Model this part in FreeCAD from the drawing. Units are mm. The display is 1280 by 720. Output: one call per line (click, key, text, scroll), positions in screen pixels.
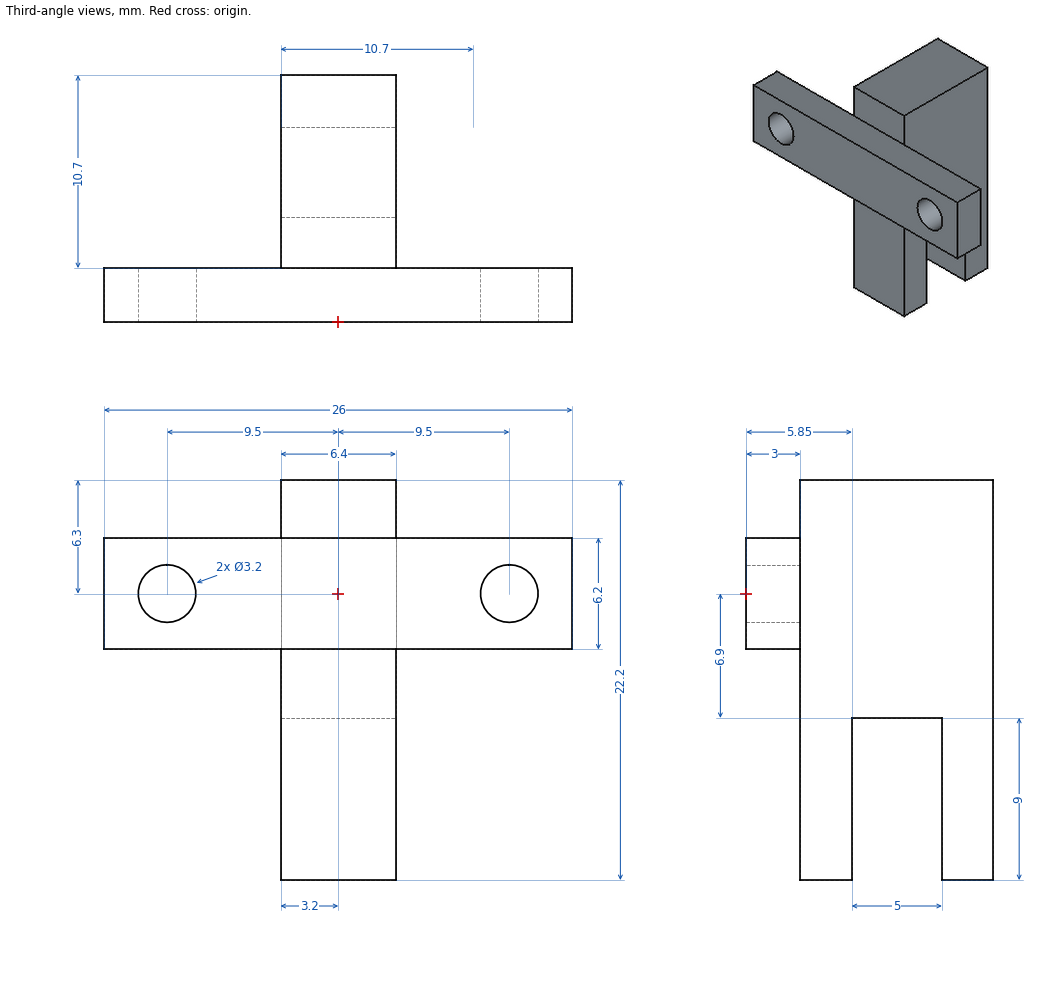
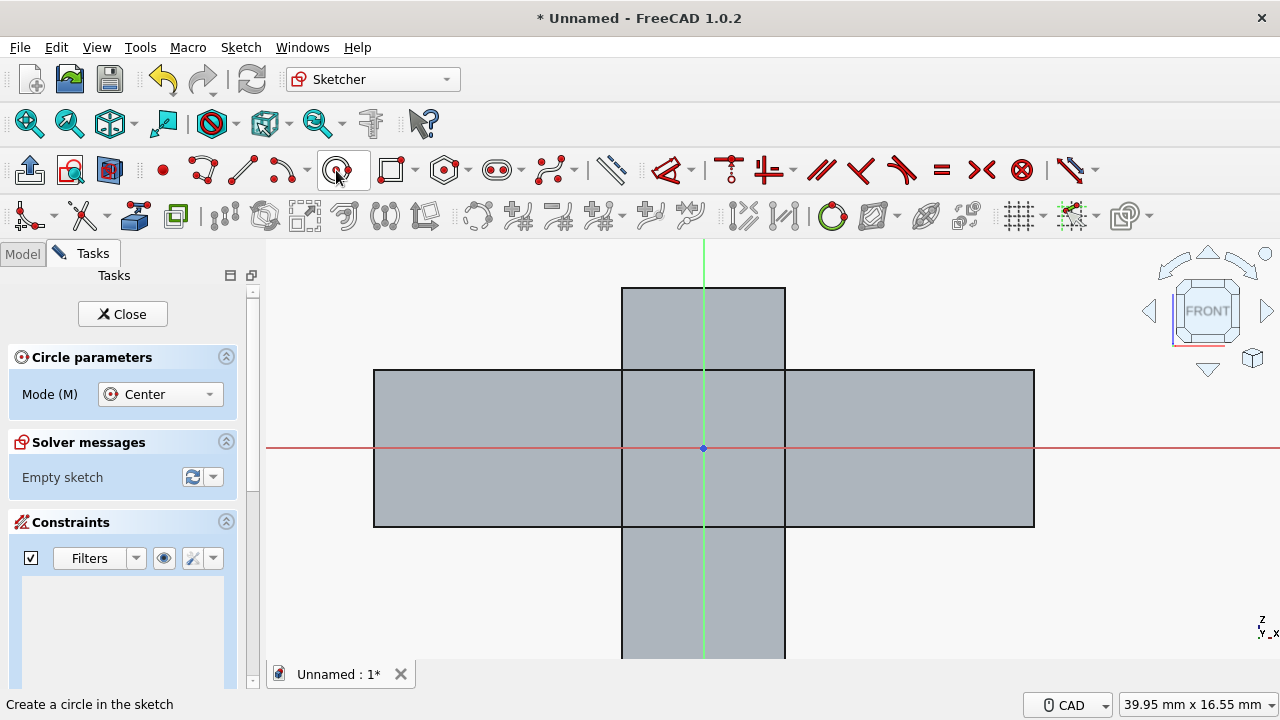
click(463, 448)
move(491, 419)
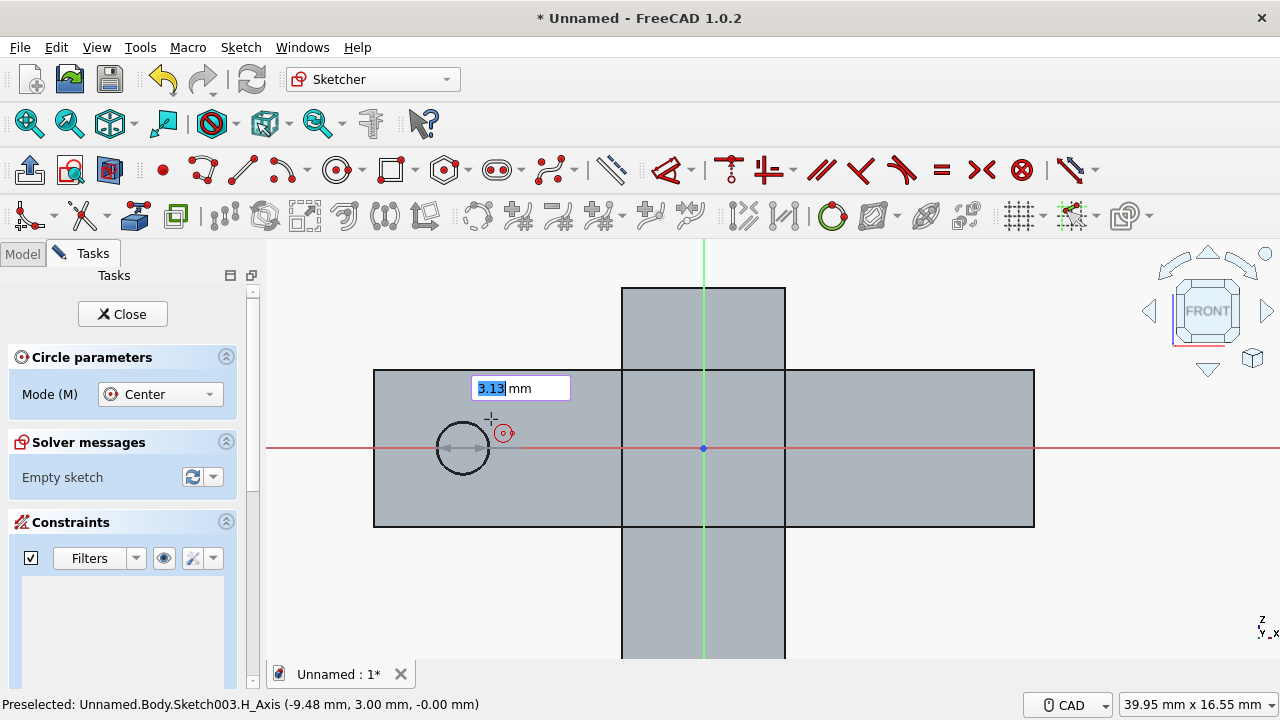
text(3.2)
key(Return)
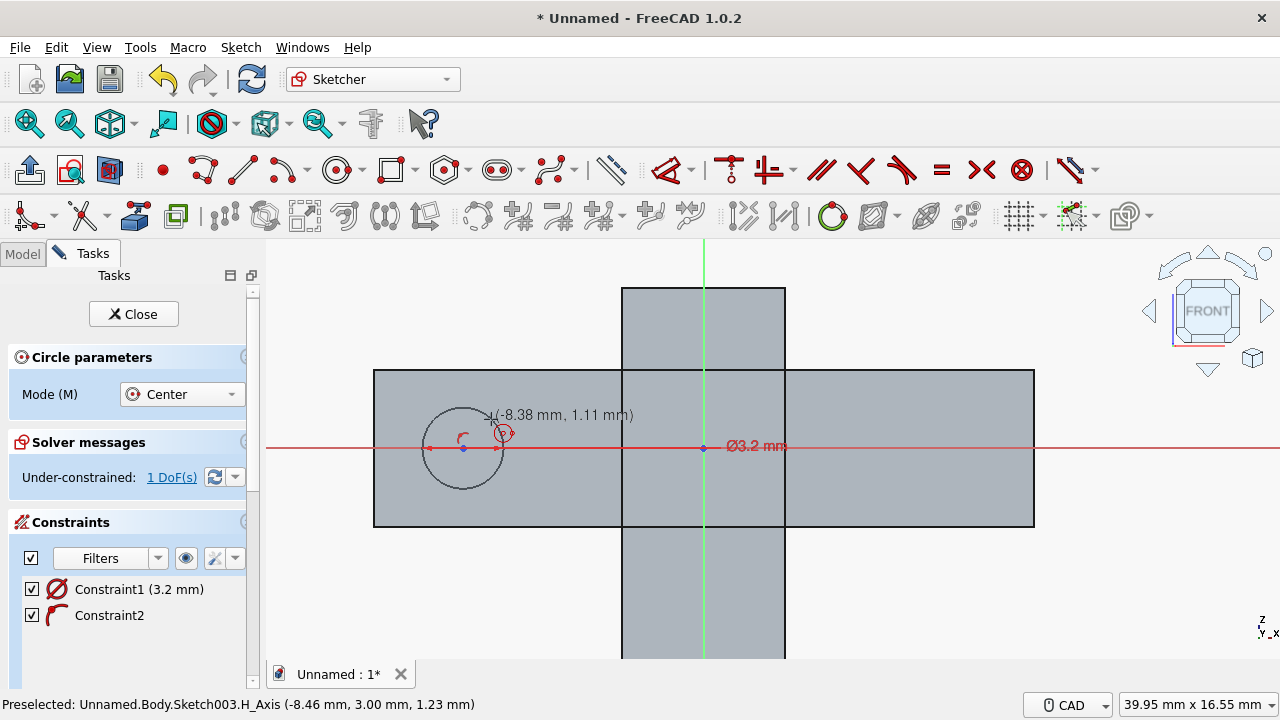
click(945, 448)
move(973, 419)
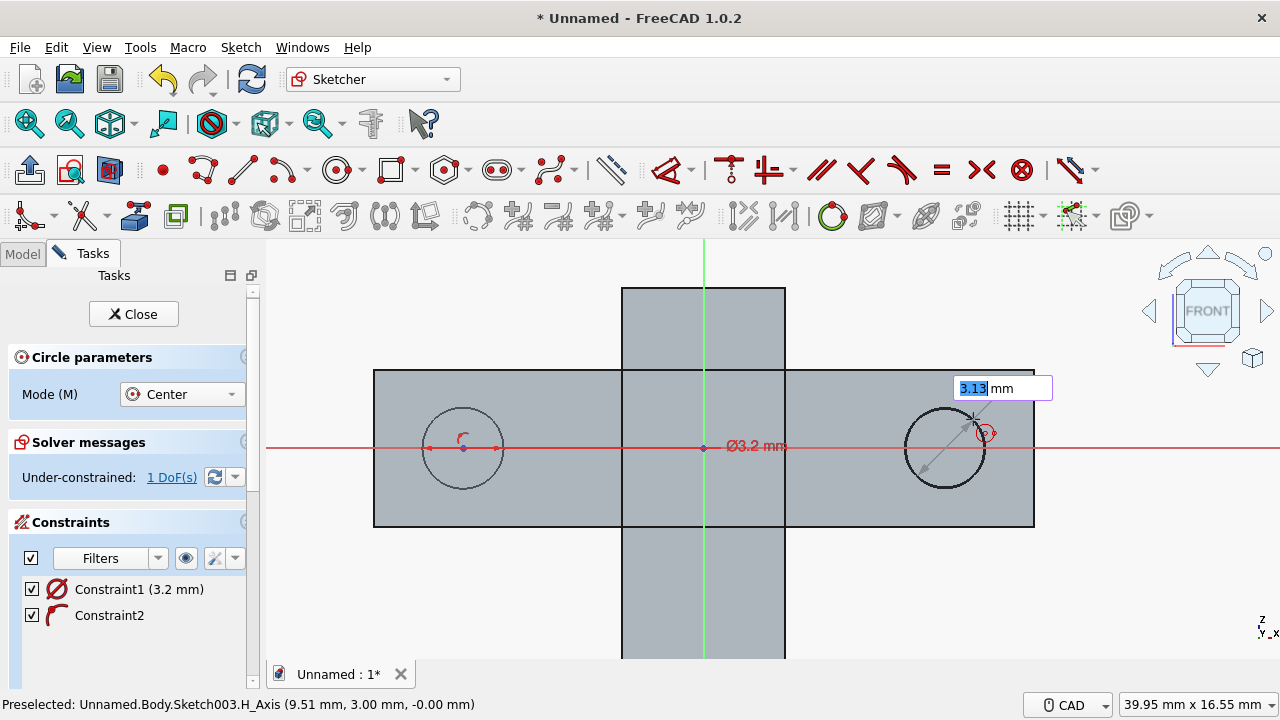
text(3.2)
key(Return)
key(Escape)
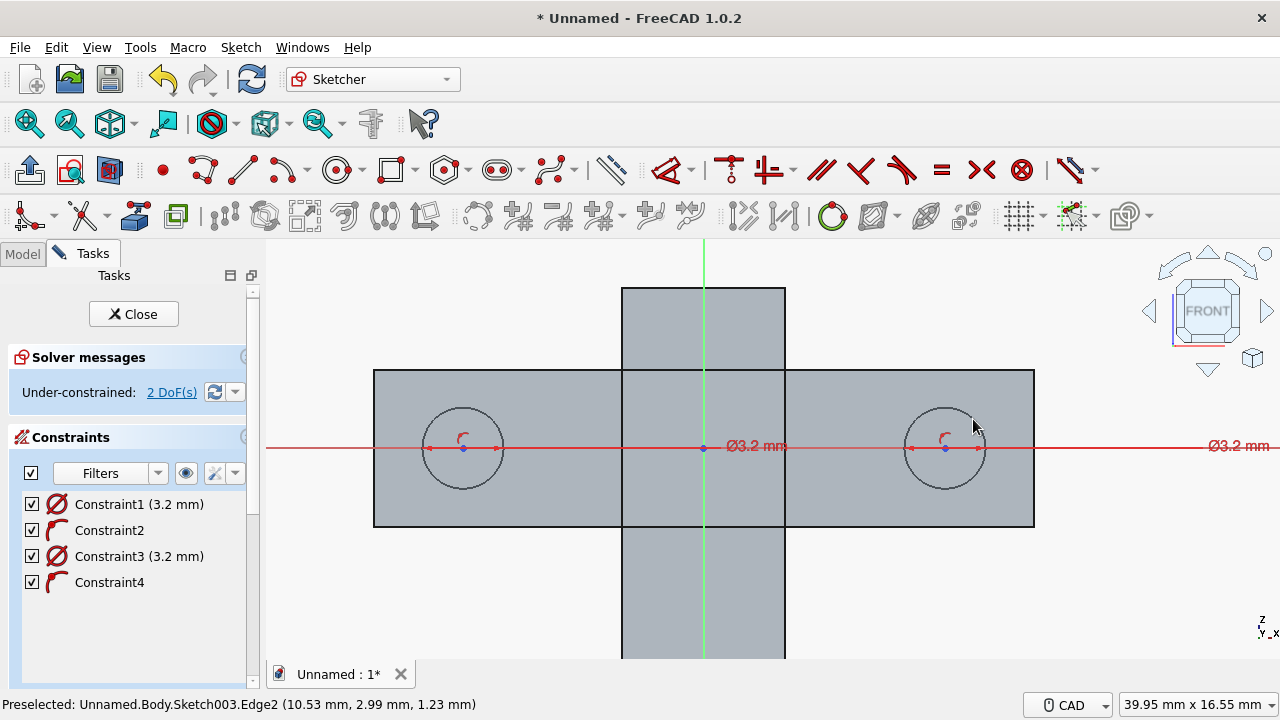
key(d)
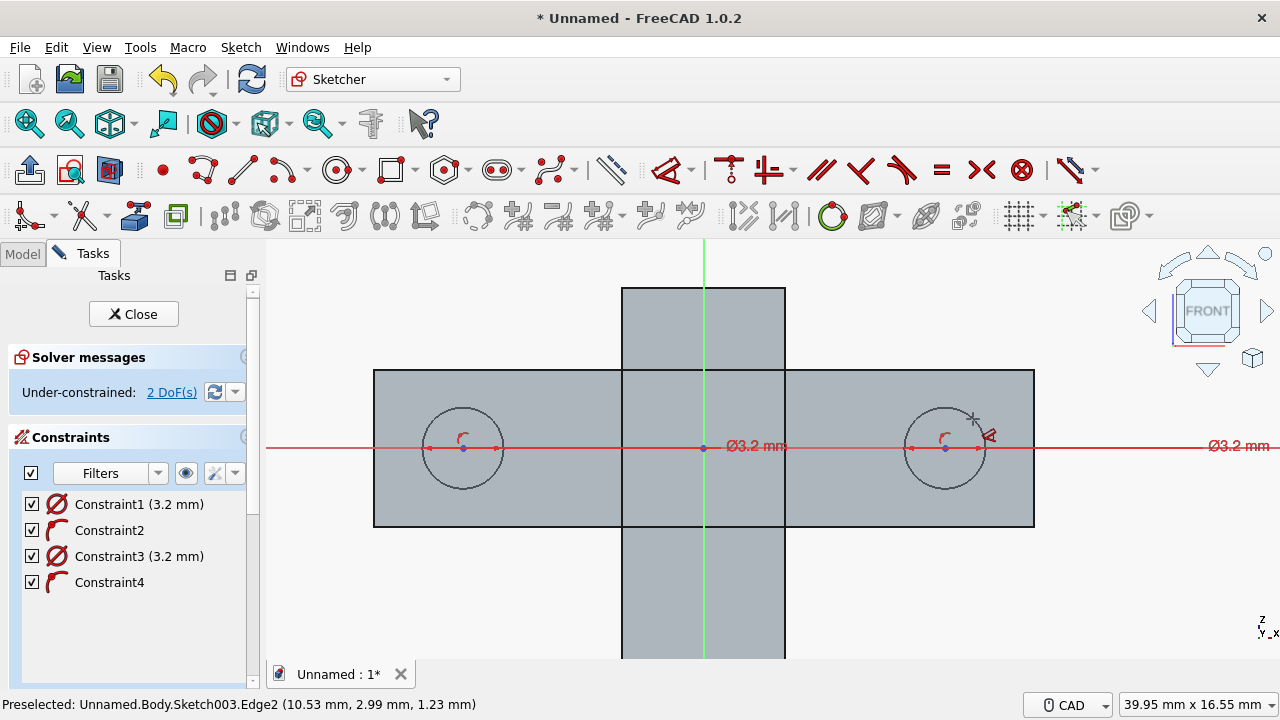
click(463, 448)
click(583, 482)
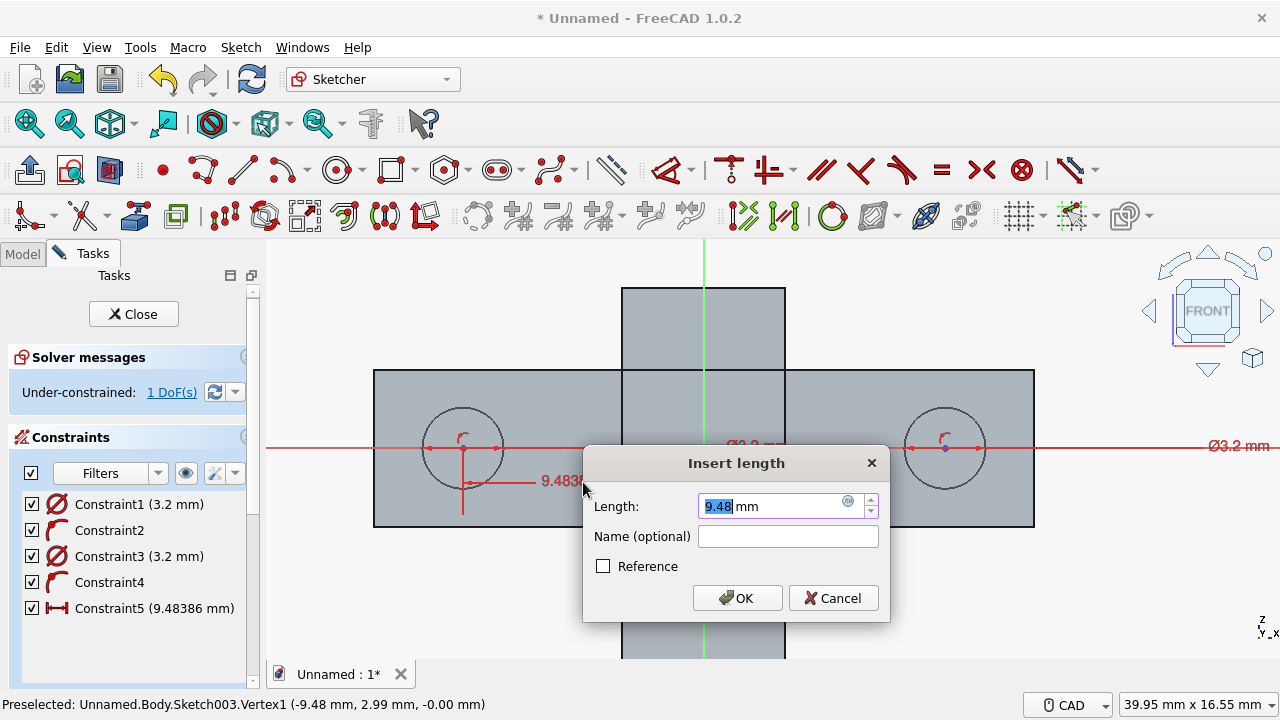
text(9.5)
key(Return)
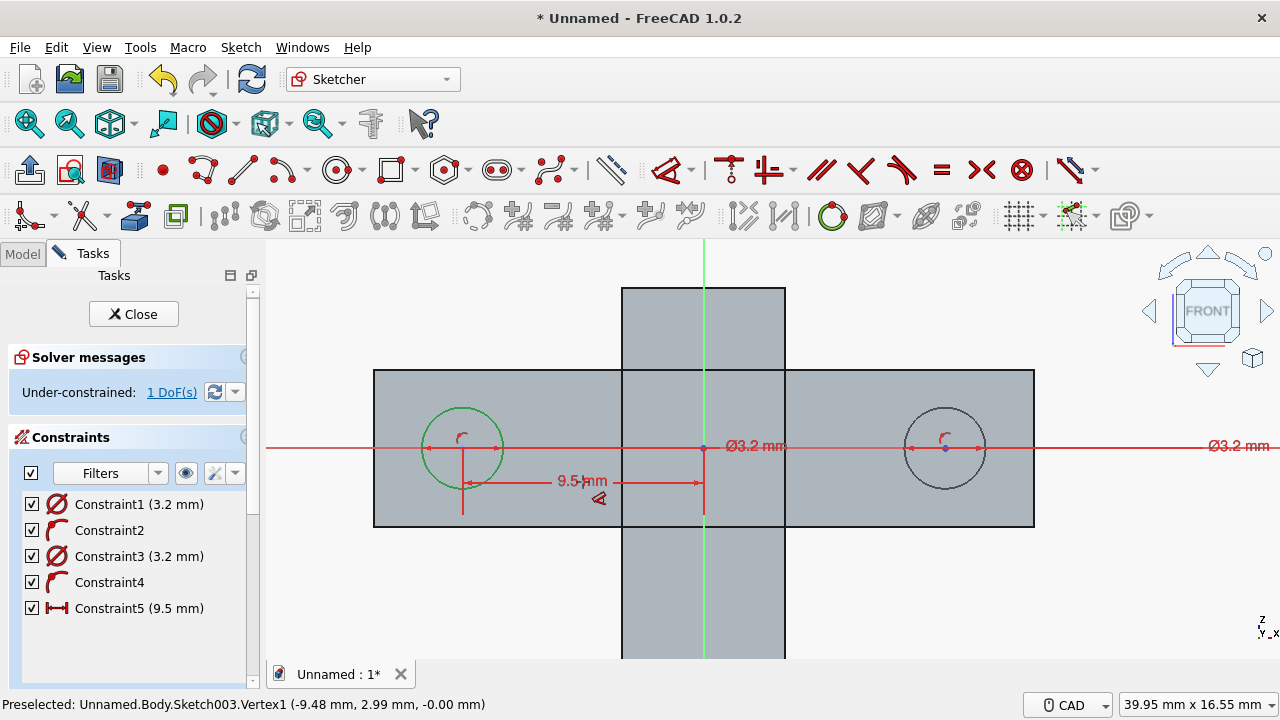
click(945, 448)
click(824, 482)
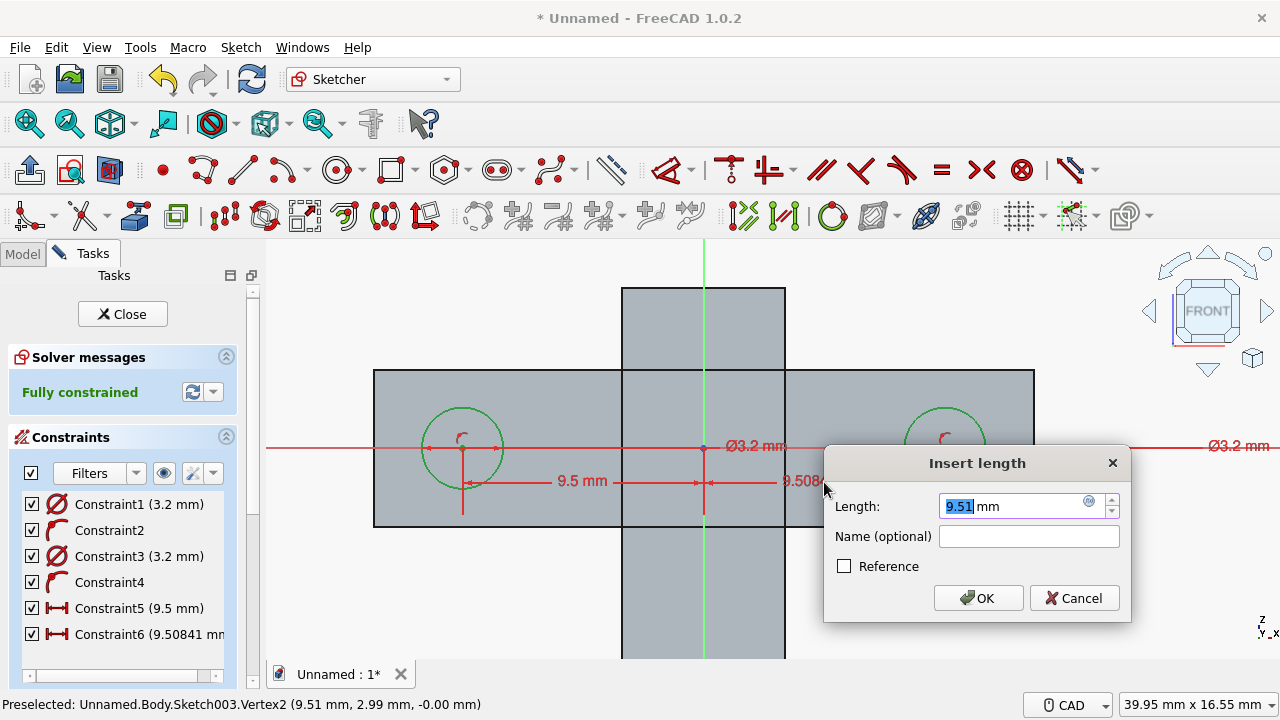
text(9.5)
key(Return)
key(Escape)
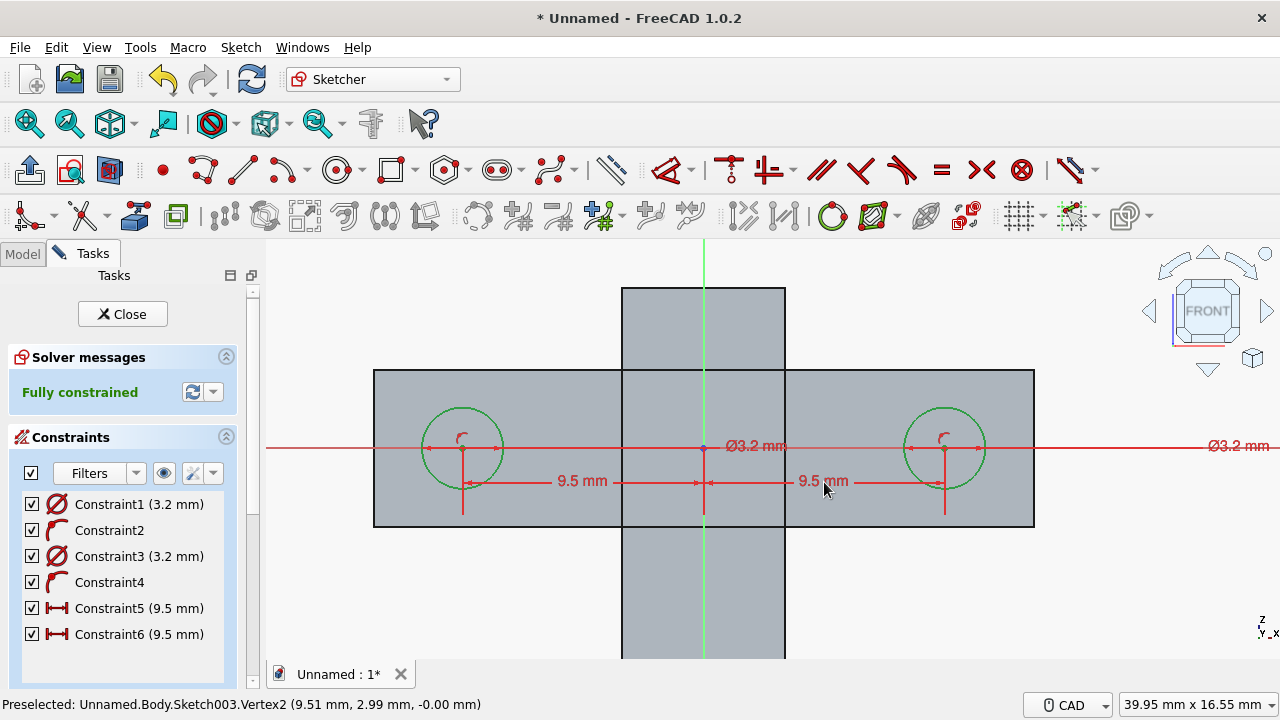
click(123, 314)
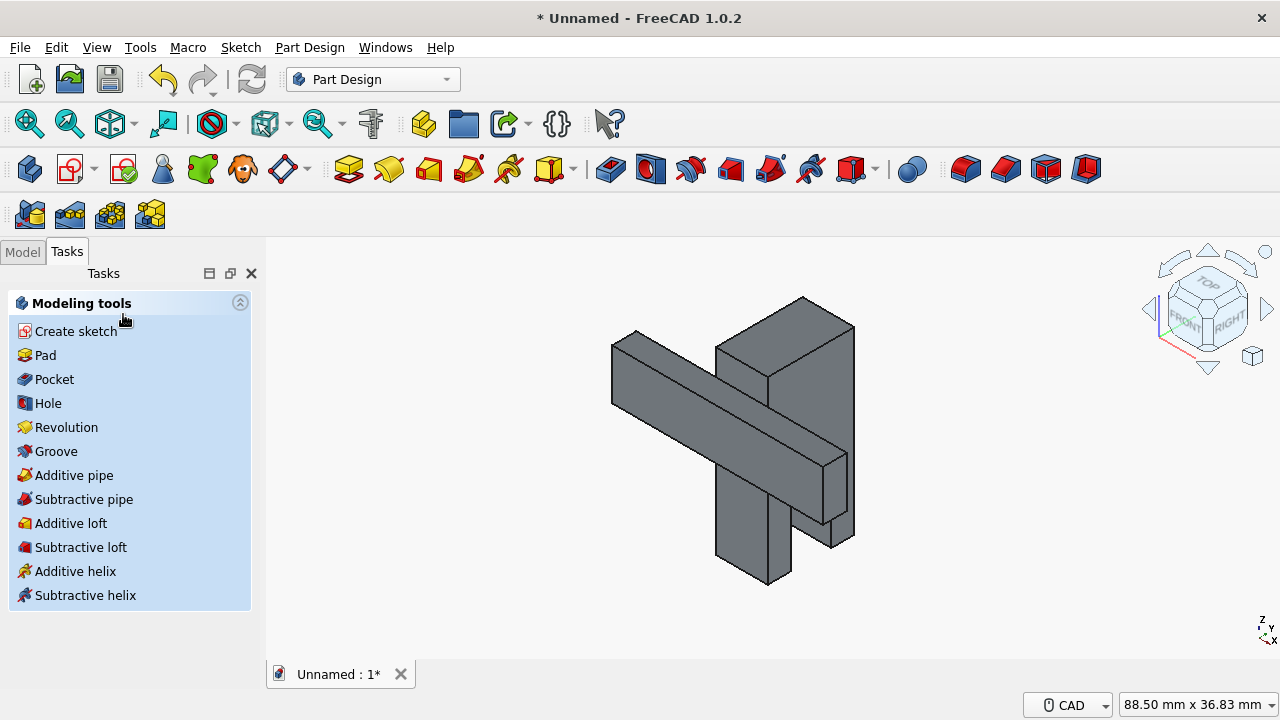
click(612, 170)